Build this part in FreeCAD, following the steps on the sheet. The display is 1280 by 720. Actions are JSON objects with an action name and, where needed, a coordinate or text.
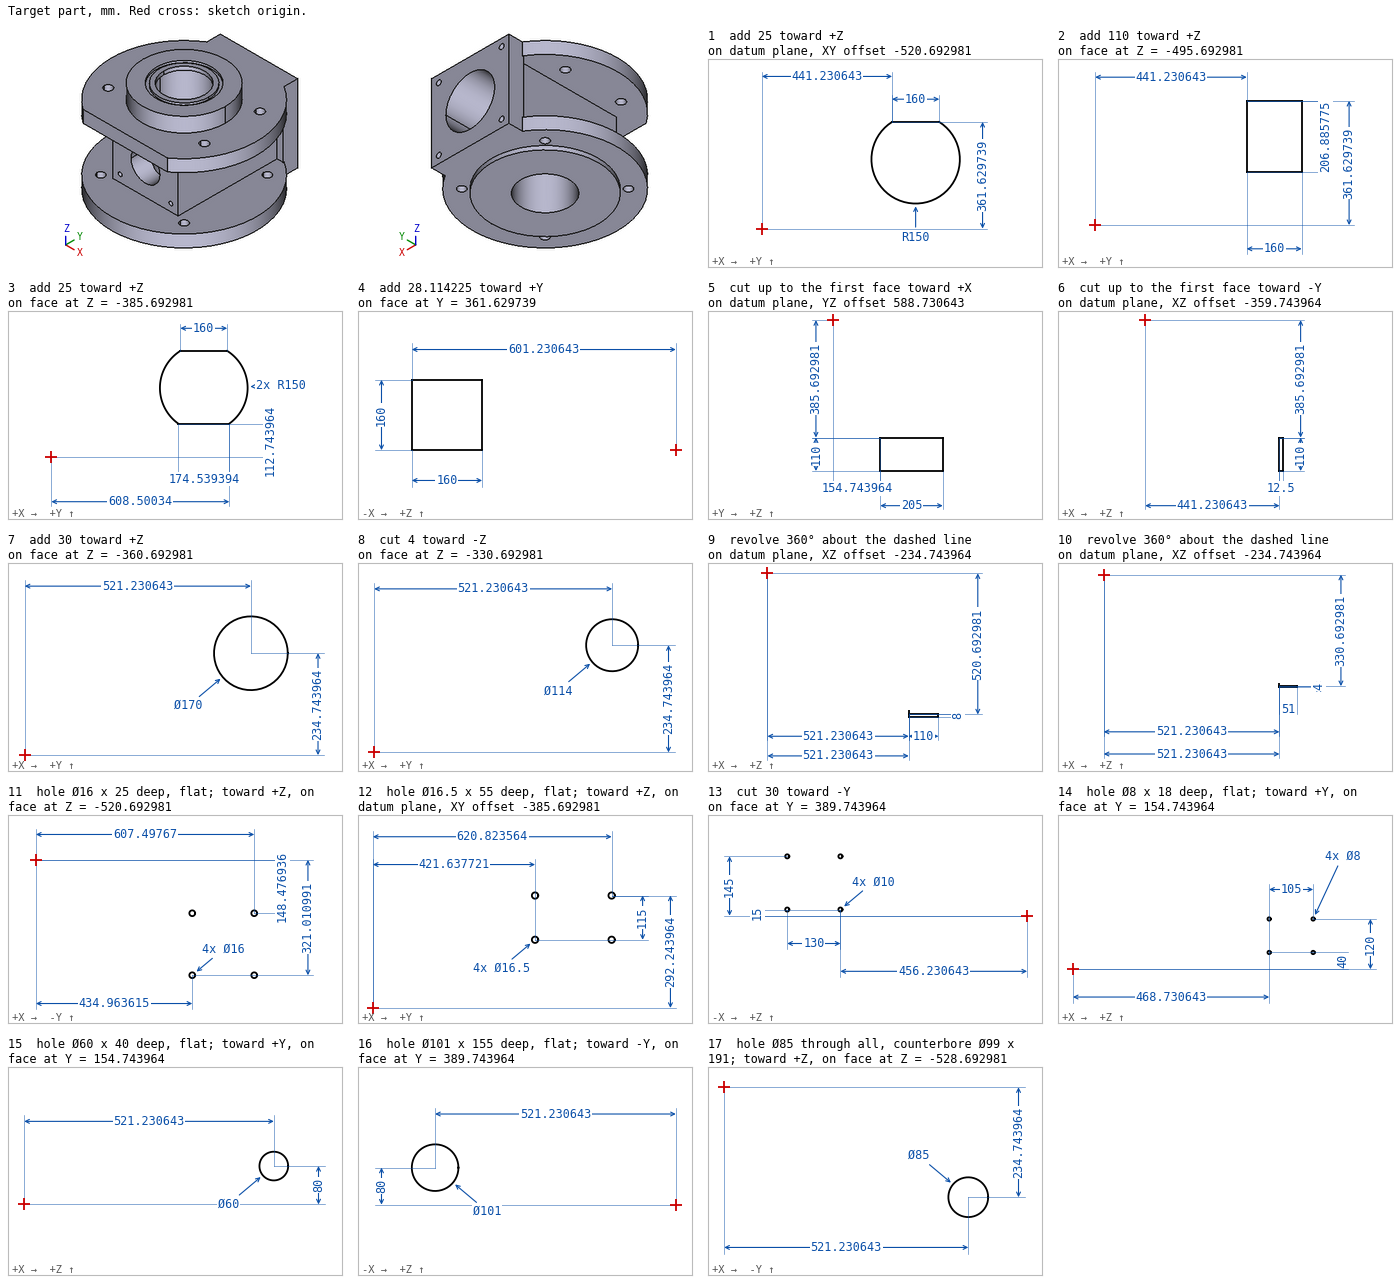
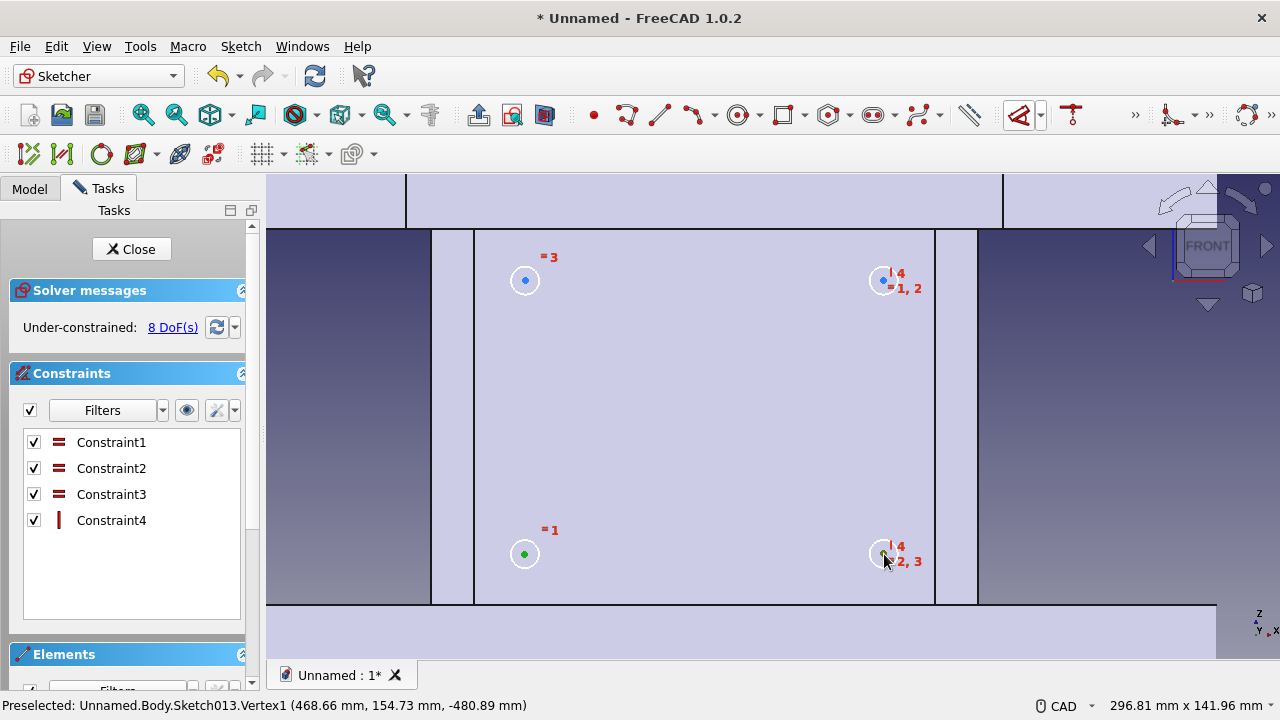
{"action": "key", "text": "h"}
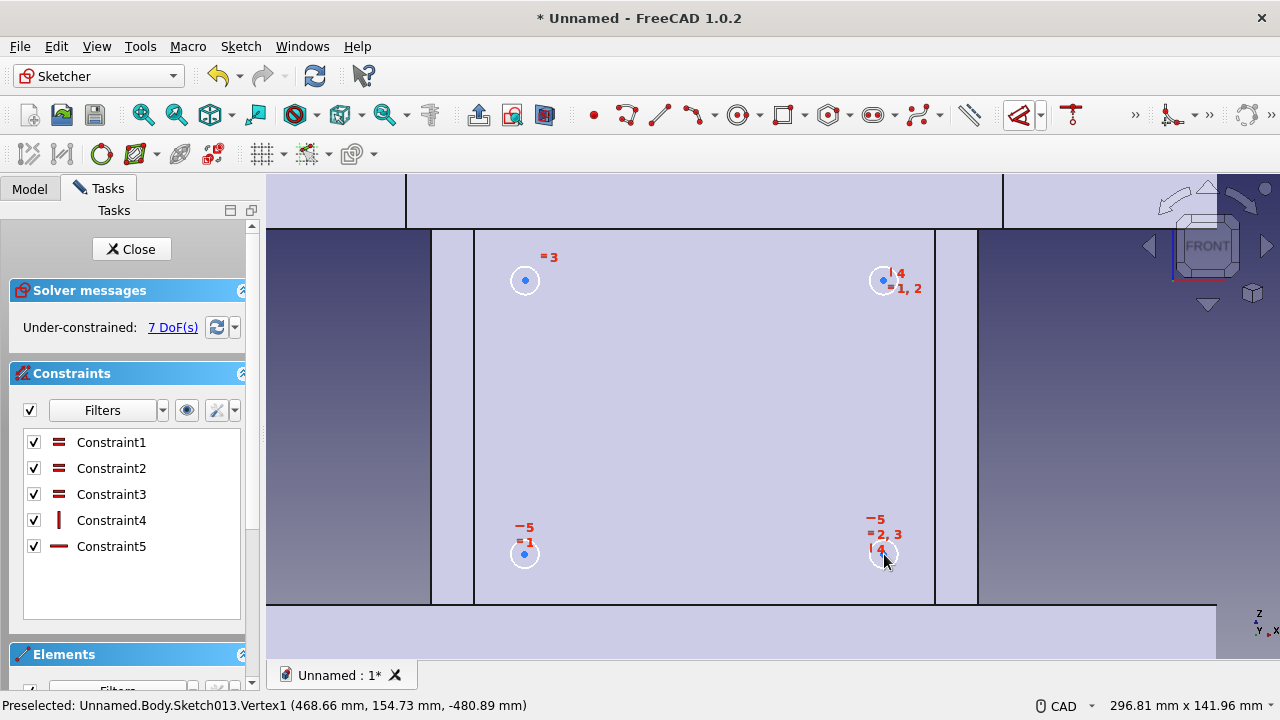
{"action": "left_click", "coordinate": [525, 554]}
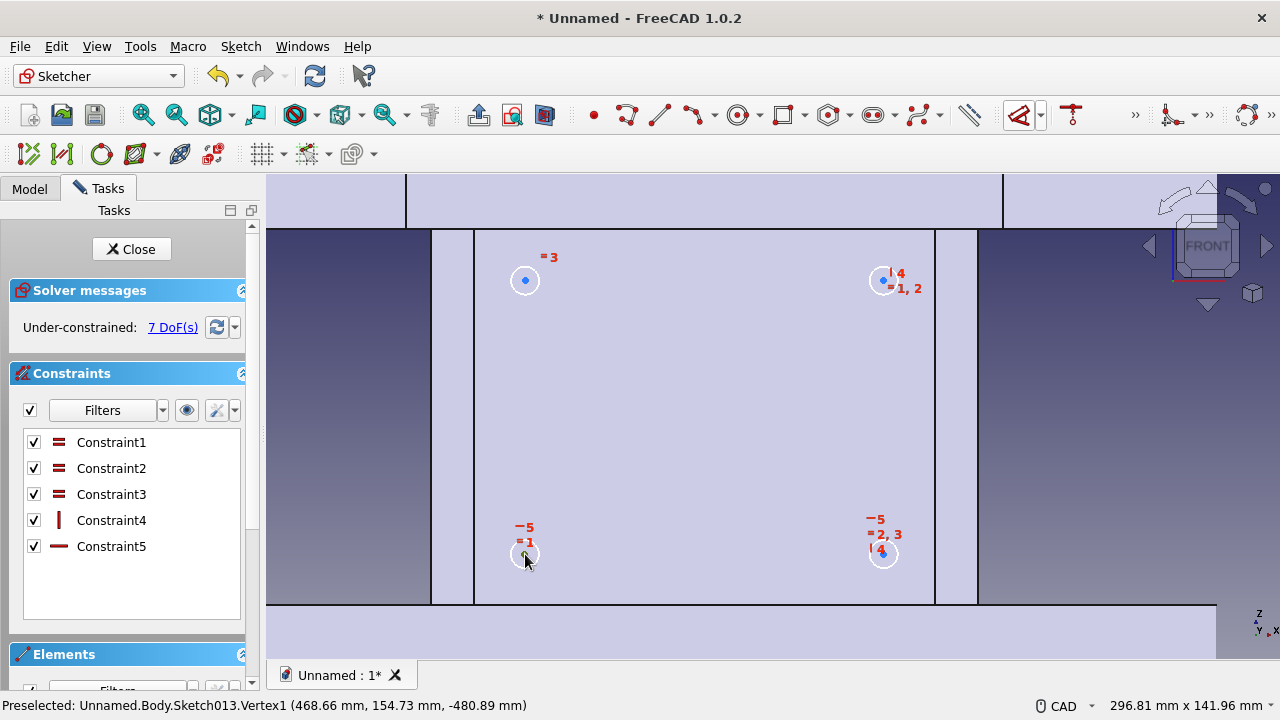
{"action": "left_click", "coordinate": [525, 281]}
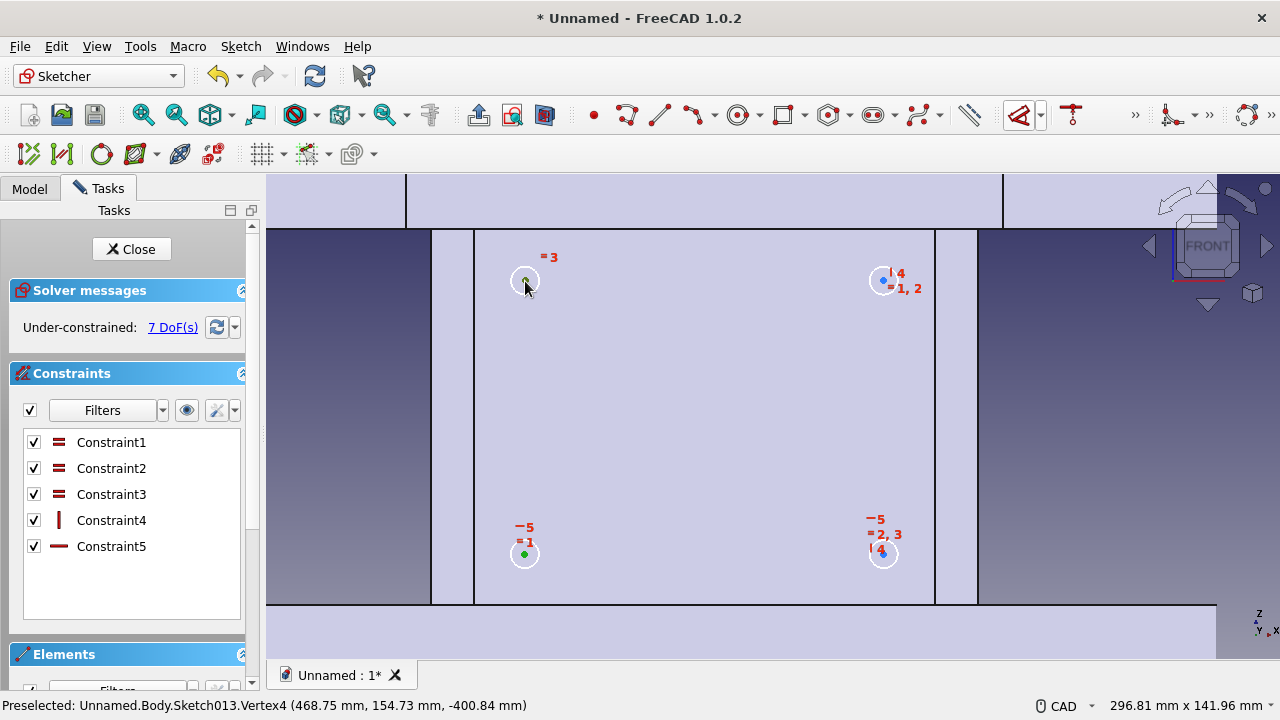
{"action": "key", "text": "v"}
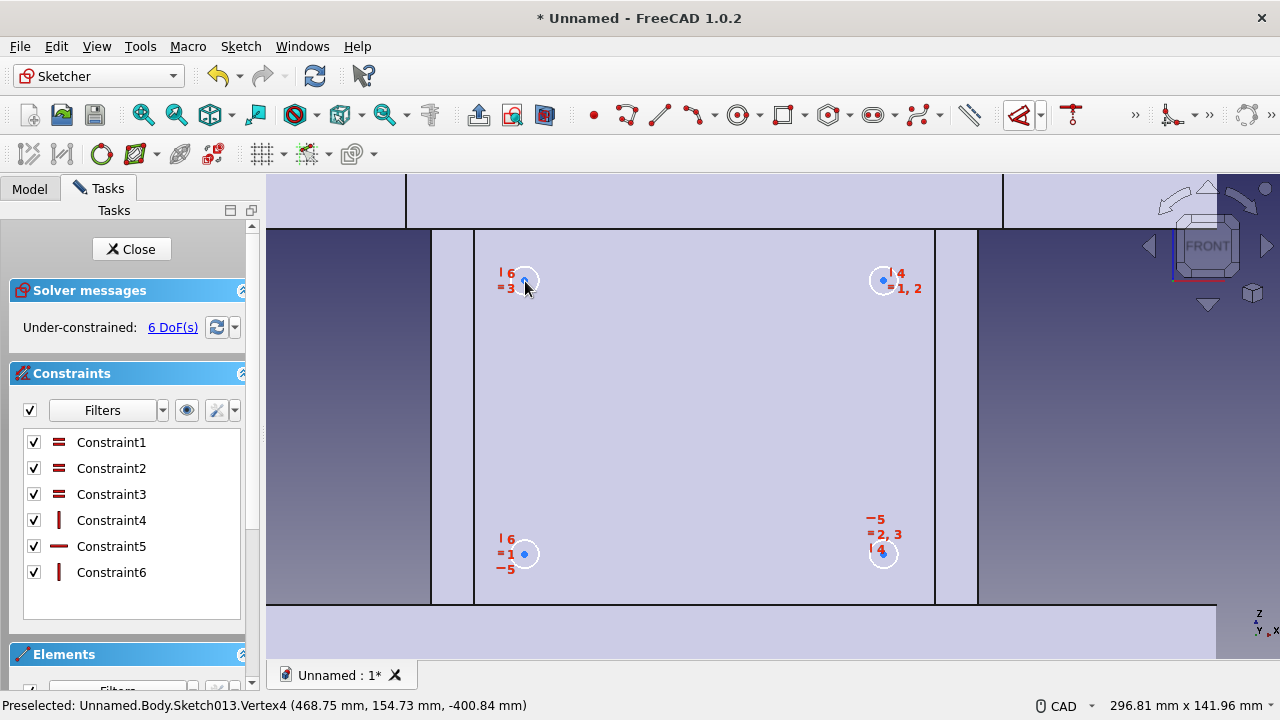
{"action": "left_click", "coordinate": [884, 281]}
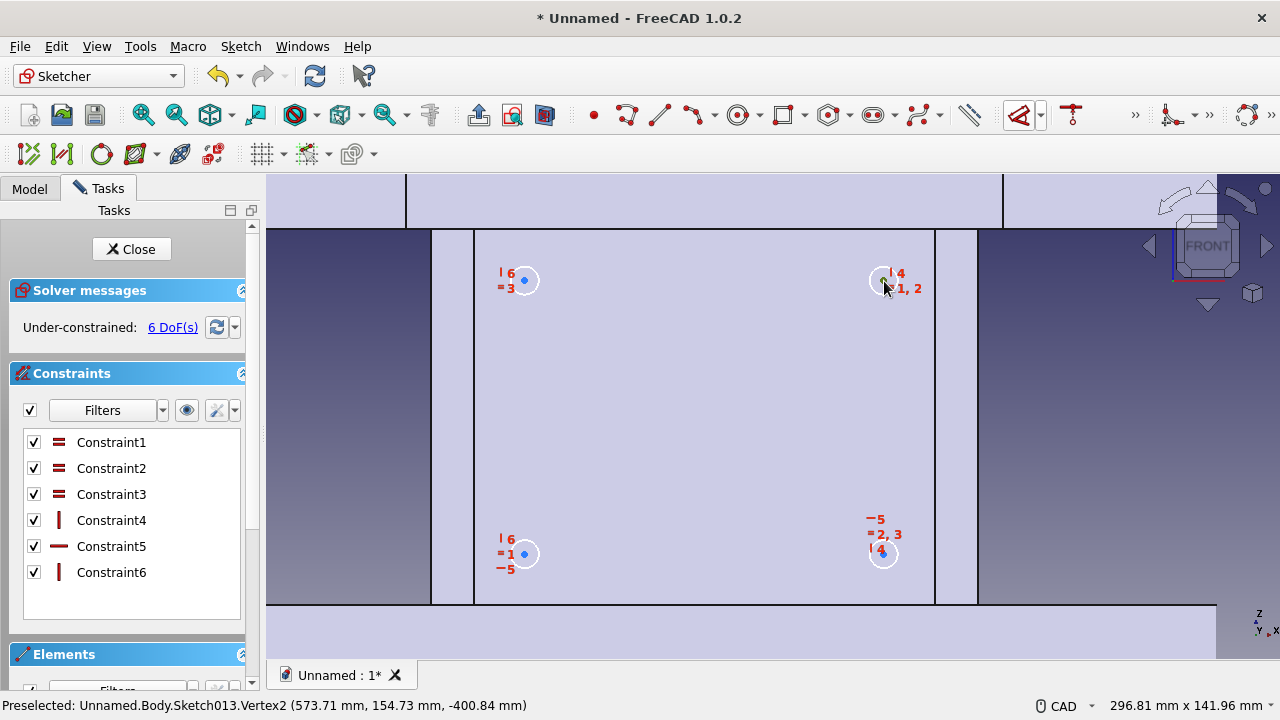
{"action": "left_click", "coordinate": [525, 281]}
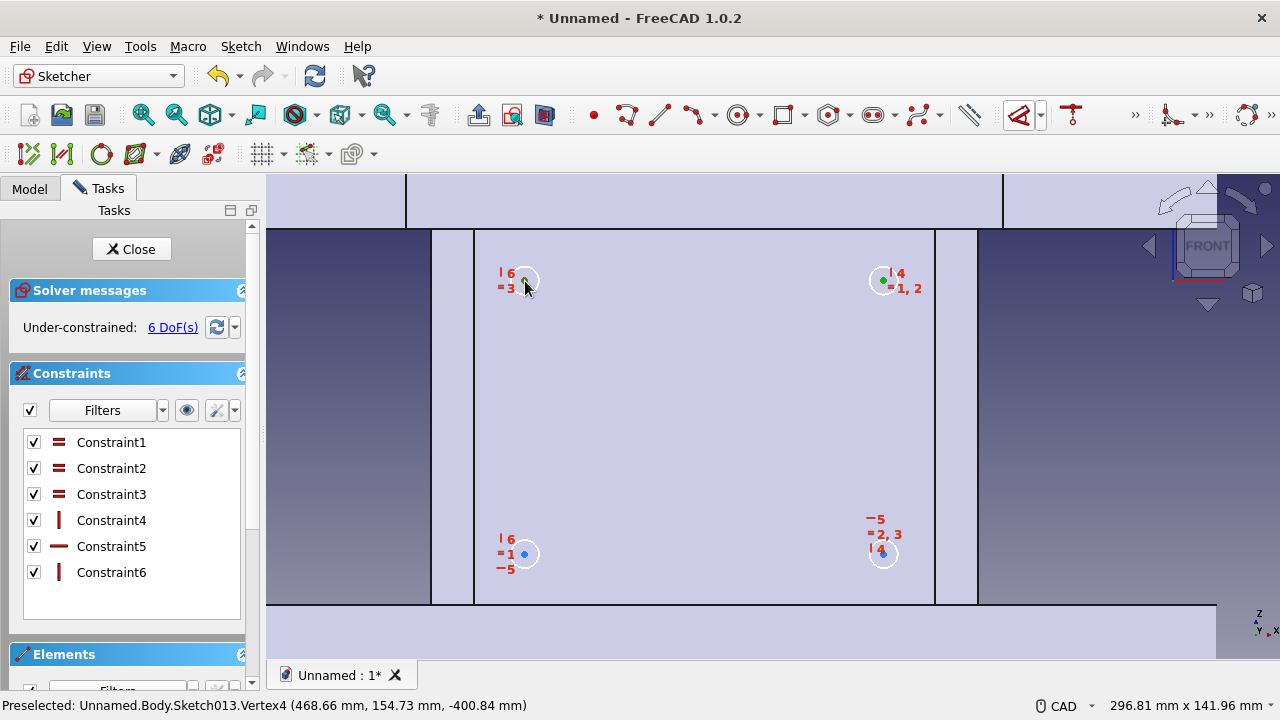
{"action": "key", "text": "h"}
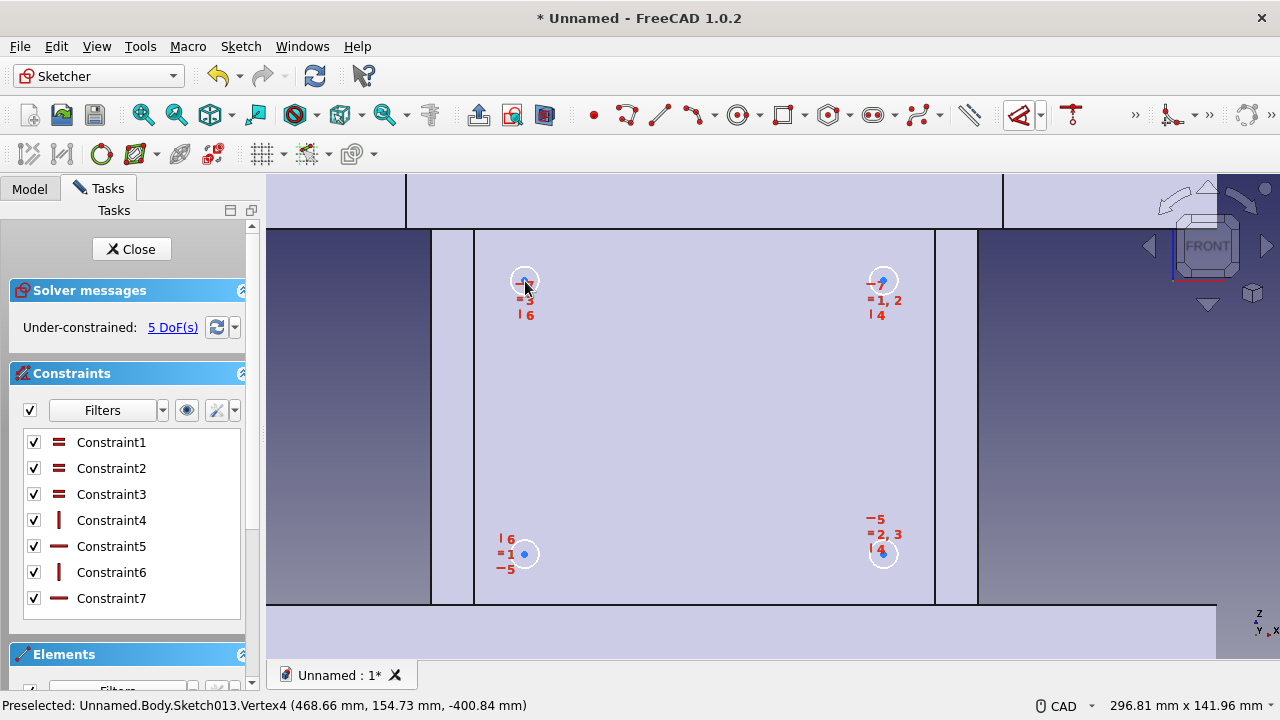
{"action": "scroll", "coordinate": [535, 544], "scroll_direction": "up", "scroll_amount": 2}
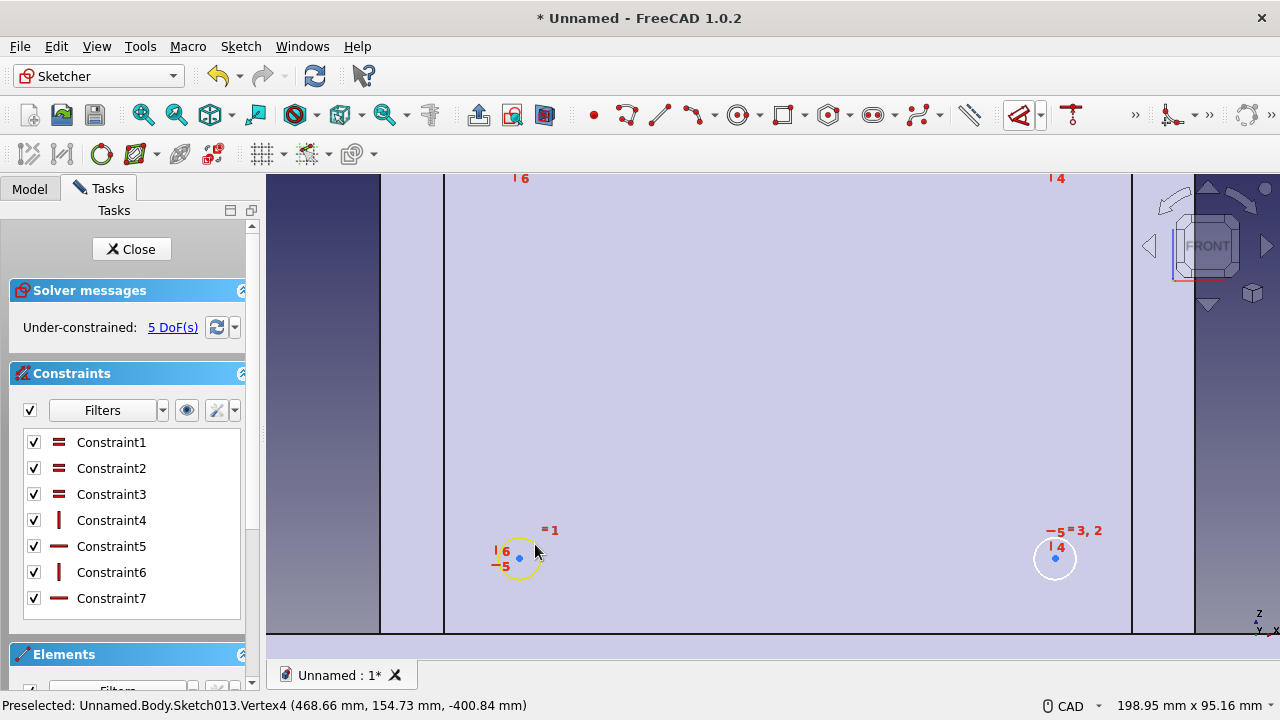
{"action": "left_click", "coordinate": [534, 544]}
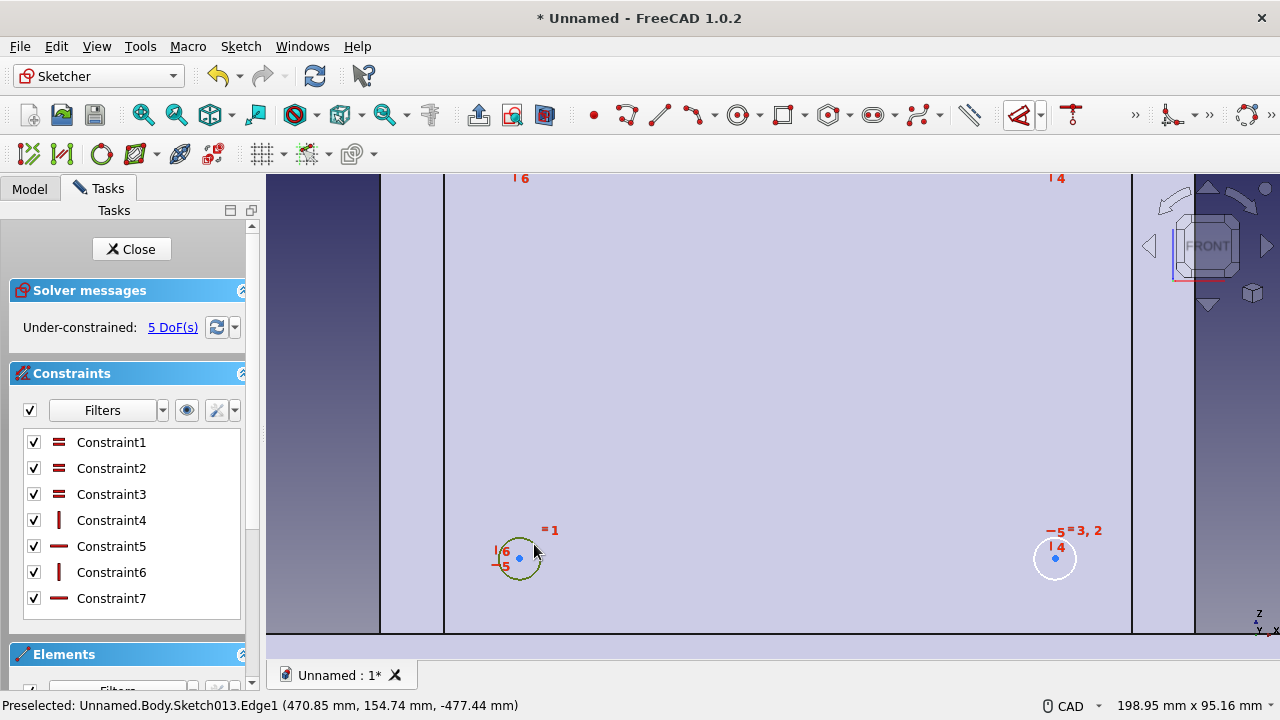
{"action": "left_click", "coordinate": [1040, 116]}